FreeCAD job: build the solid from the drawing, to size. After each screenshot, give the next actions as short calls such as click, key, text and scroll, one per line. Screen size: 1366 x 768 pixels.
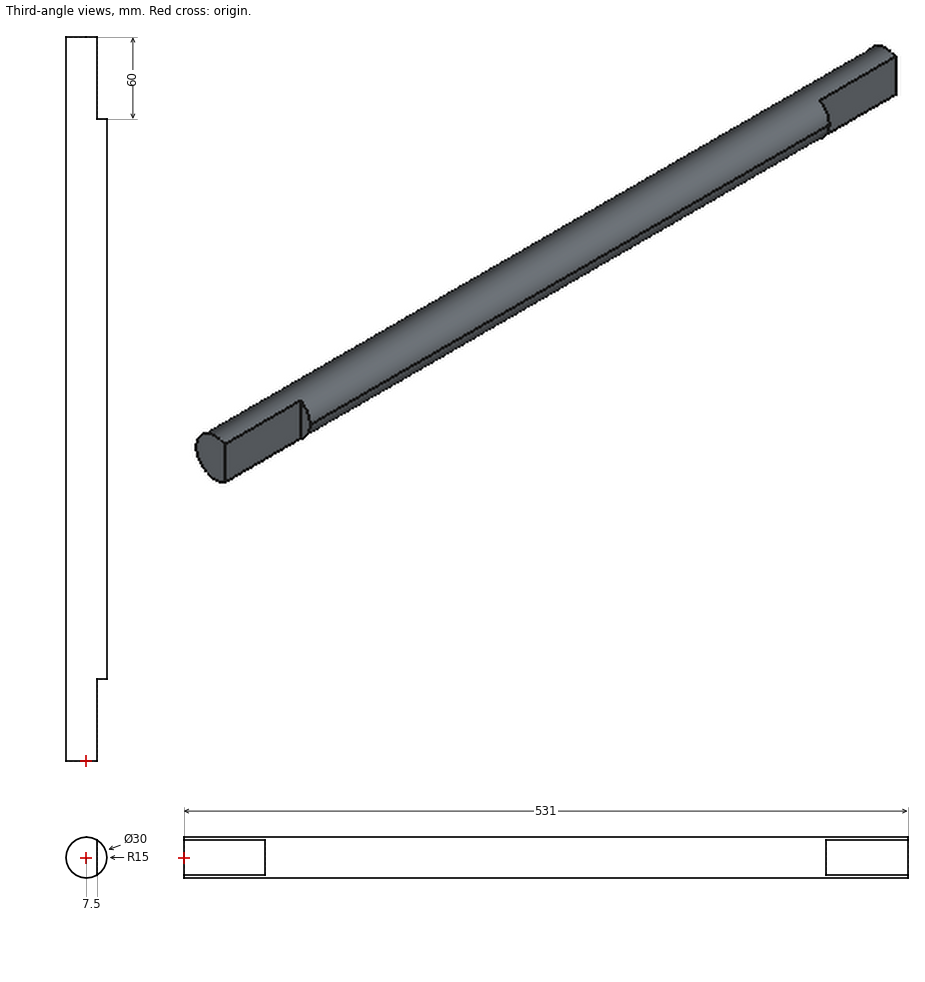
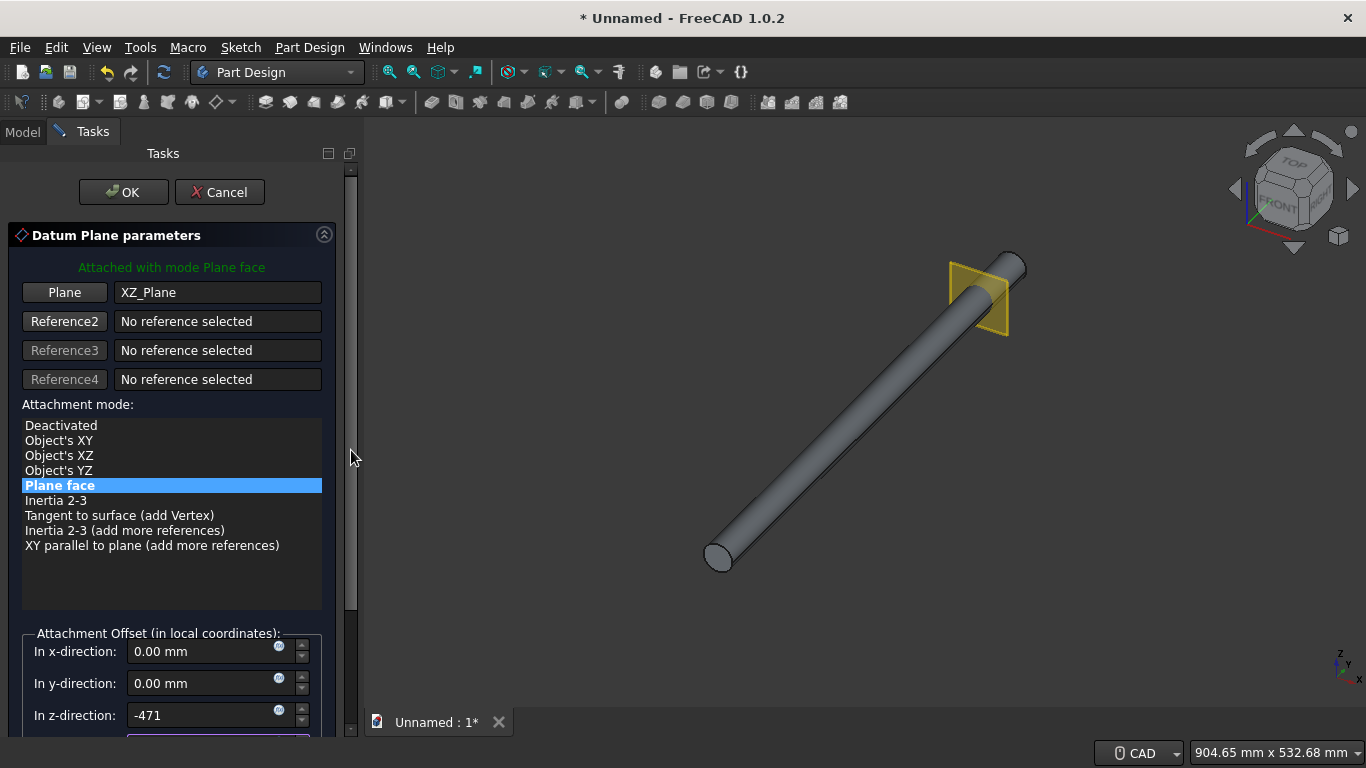
click(124, 192)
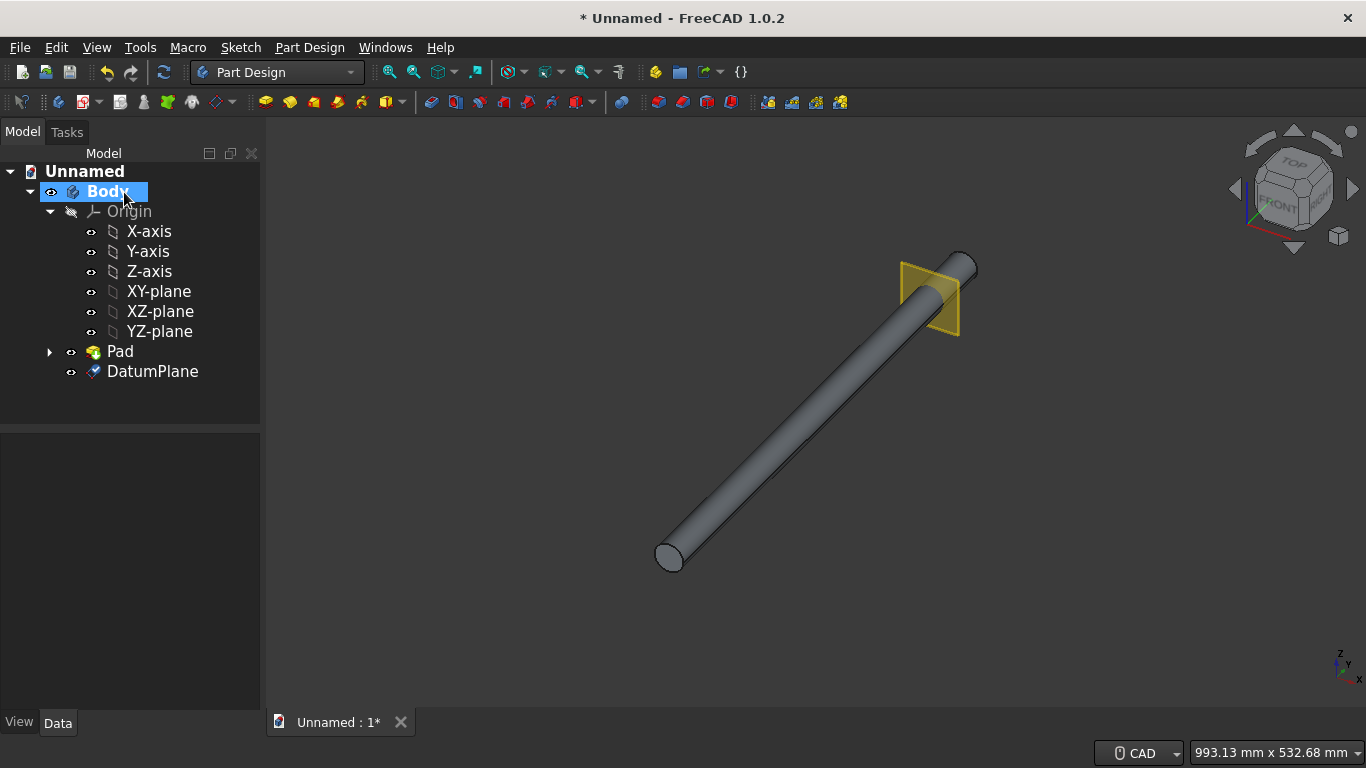
click(116, 372)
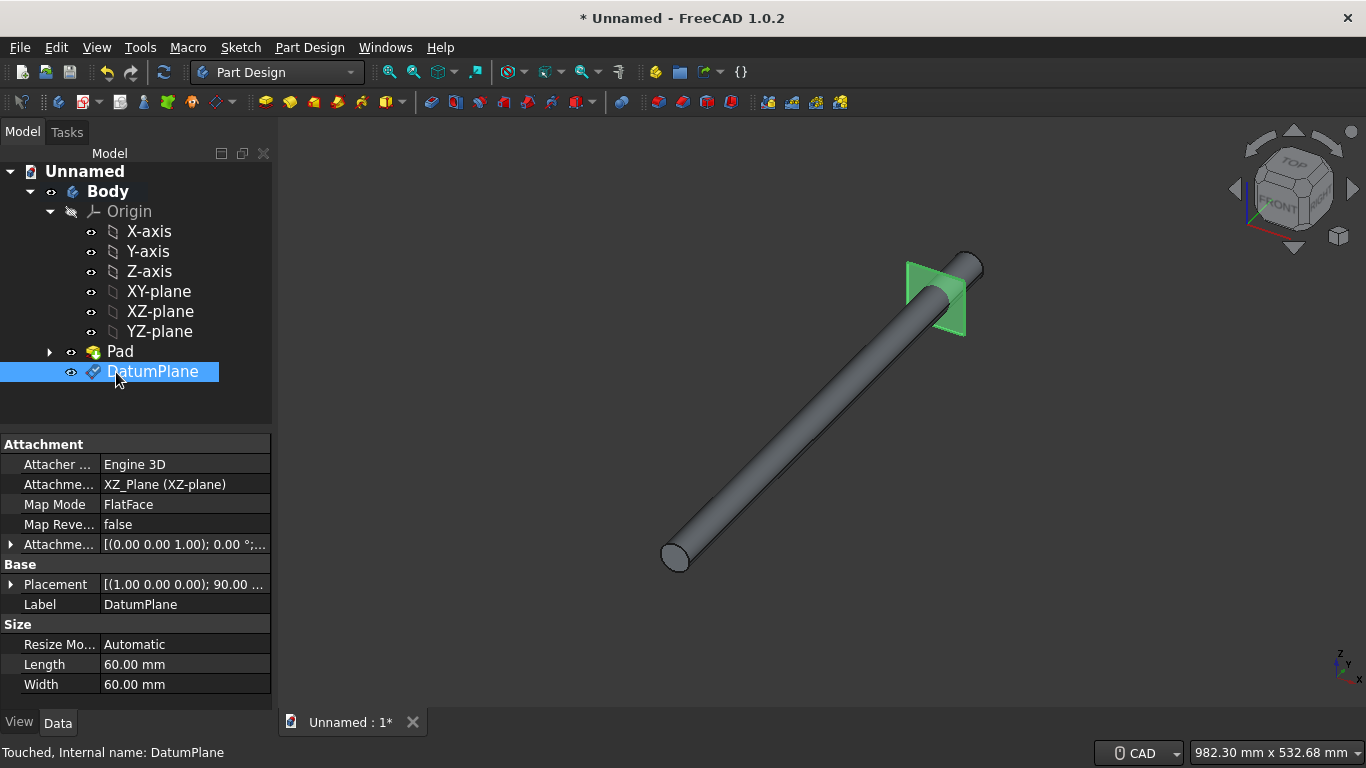
click(84, 102)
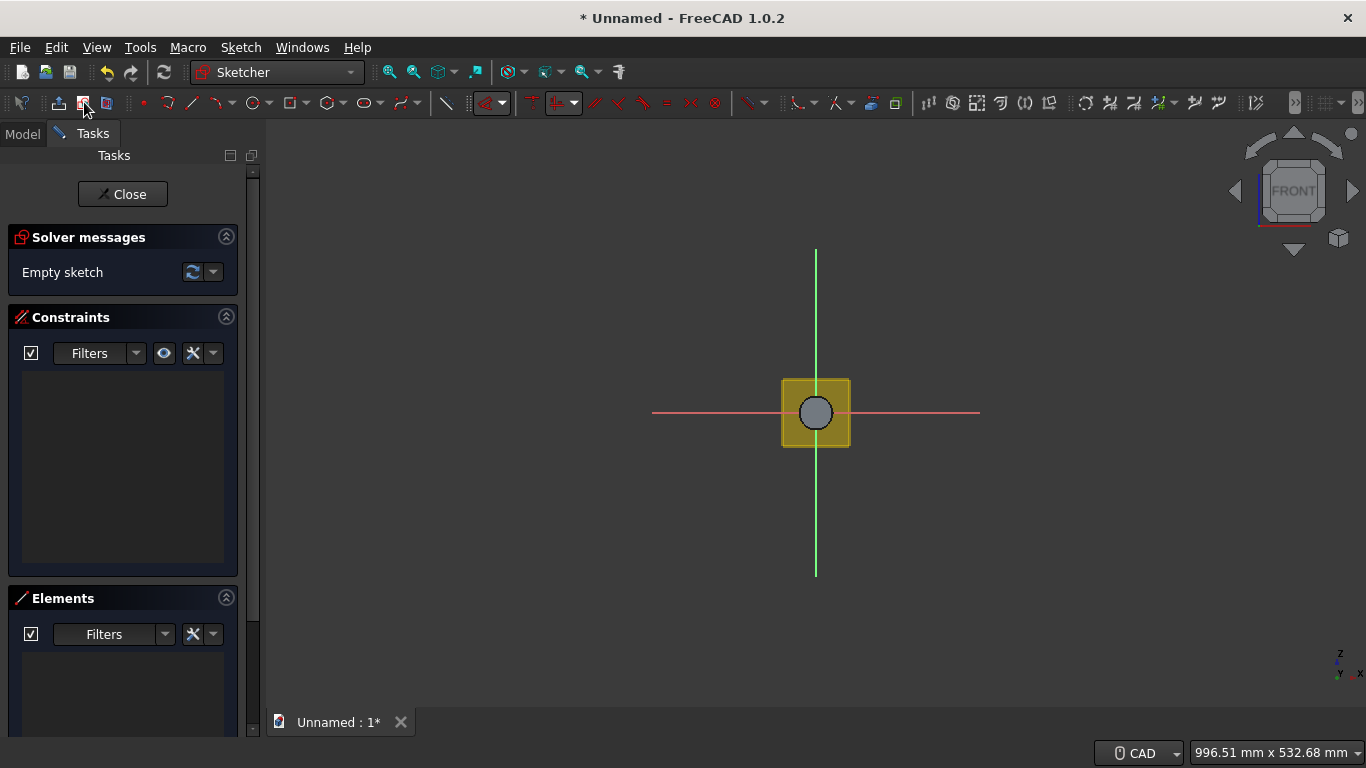
click(108, 104)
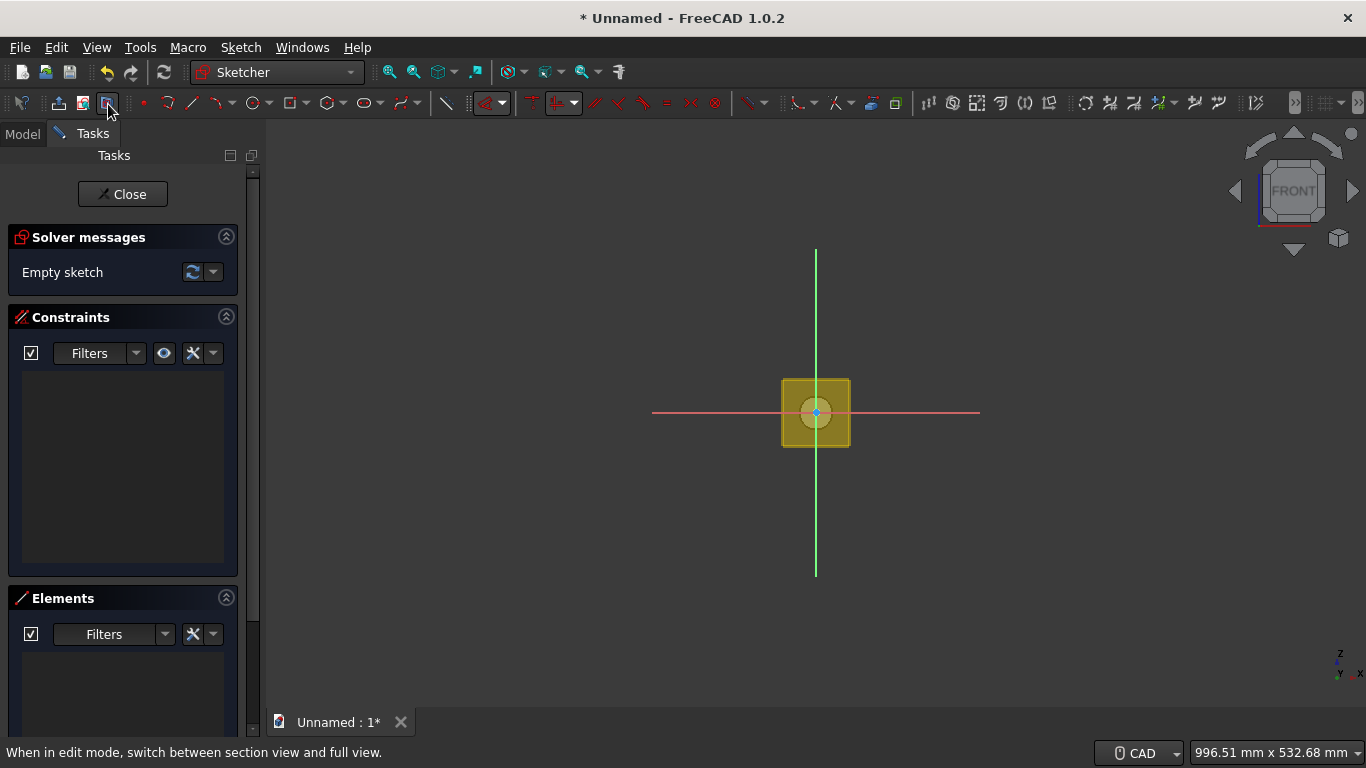
scroll(830, 413, up, 13)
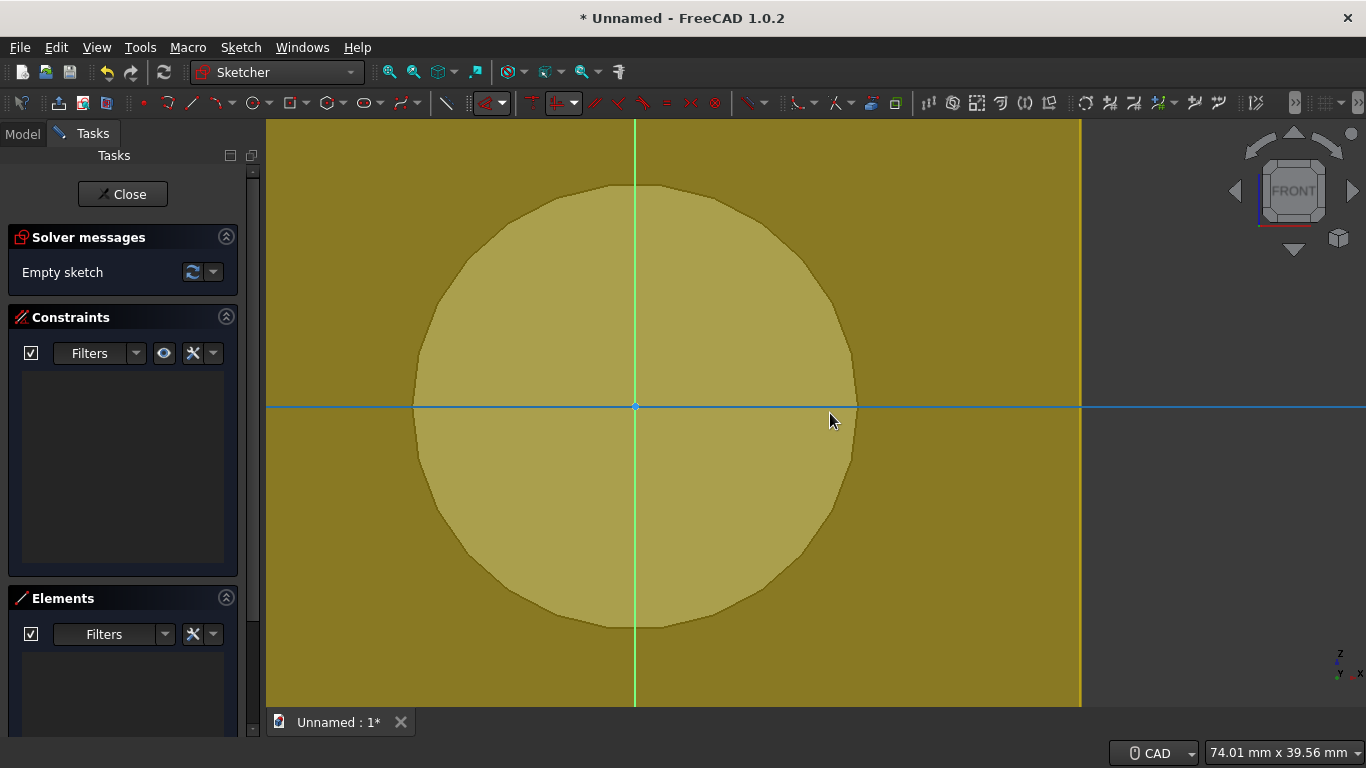
click(192, 104)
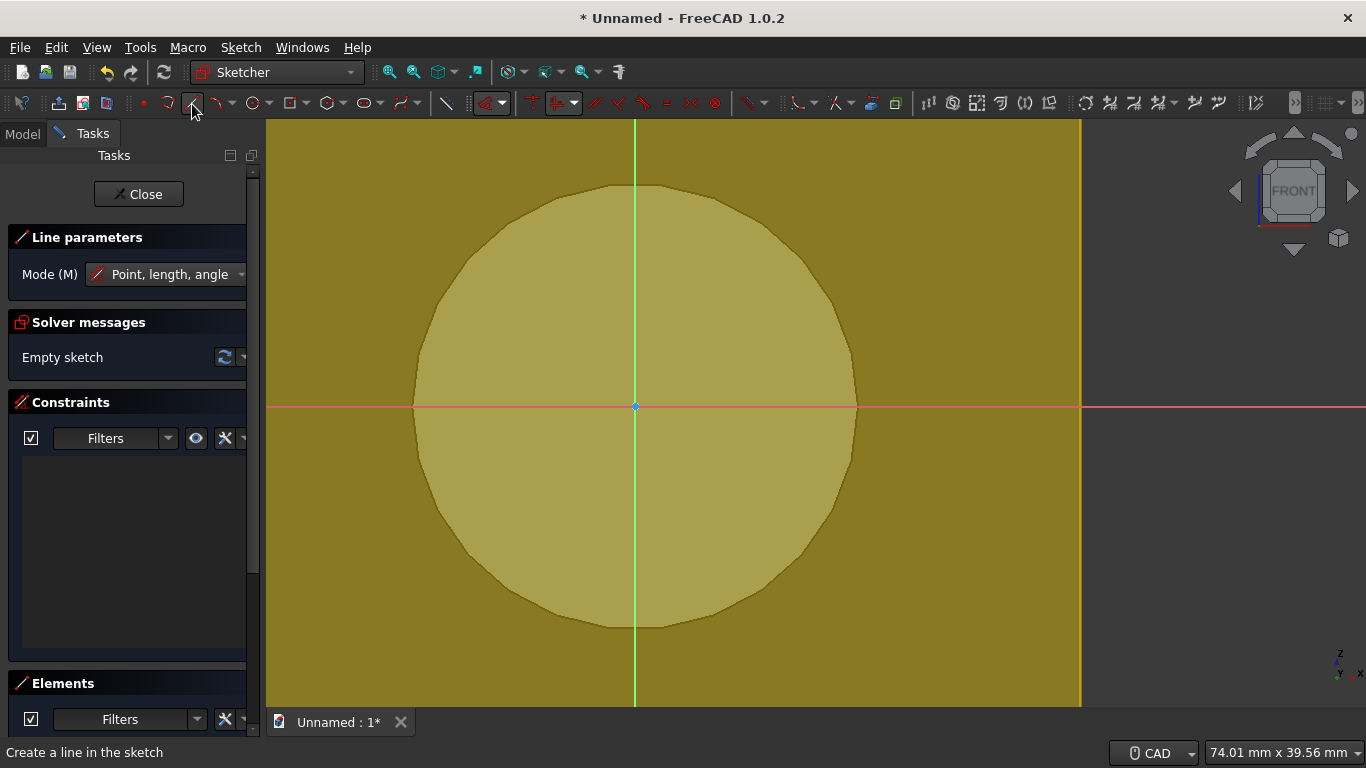
click(747, 600)
click(747, 214)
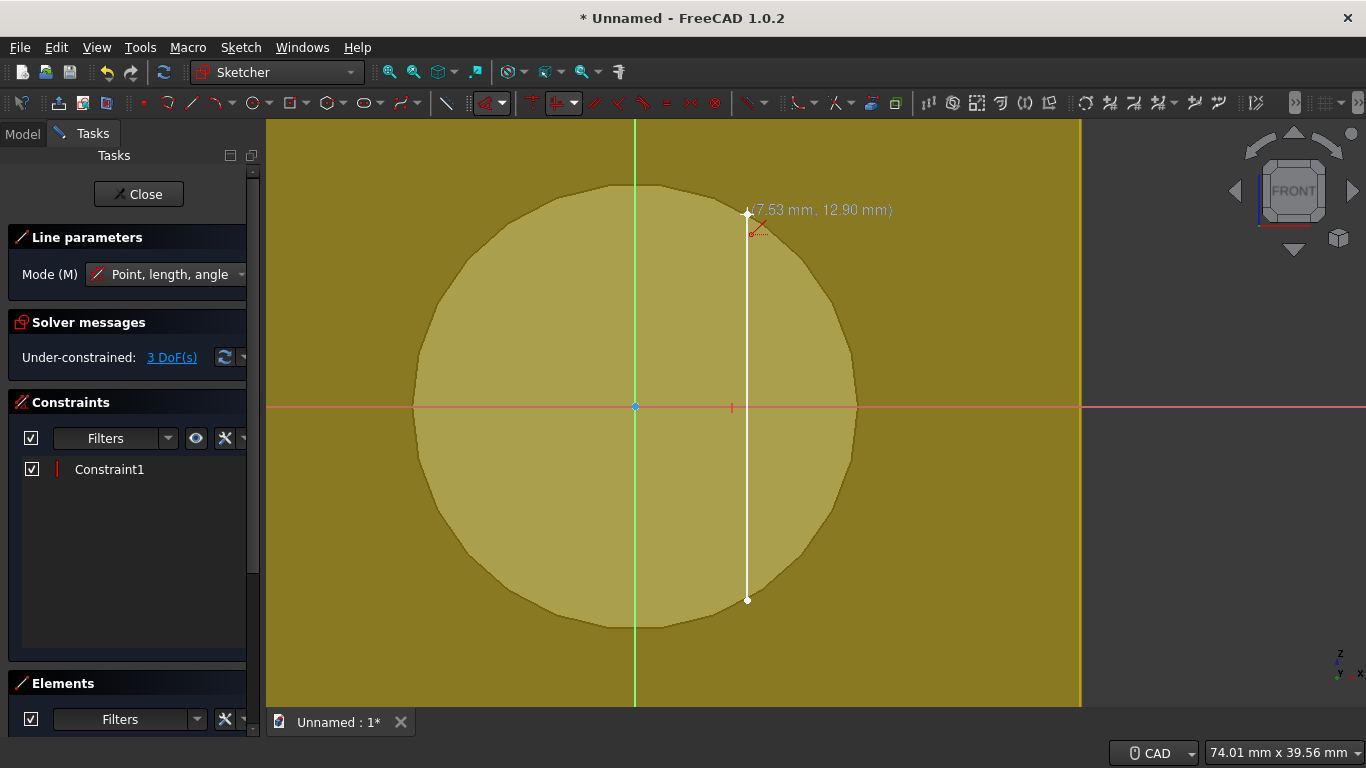
key(g)
key(3)
key(a)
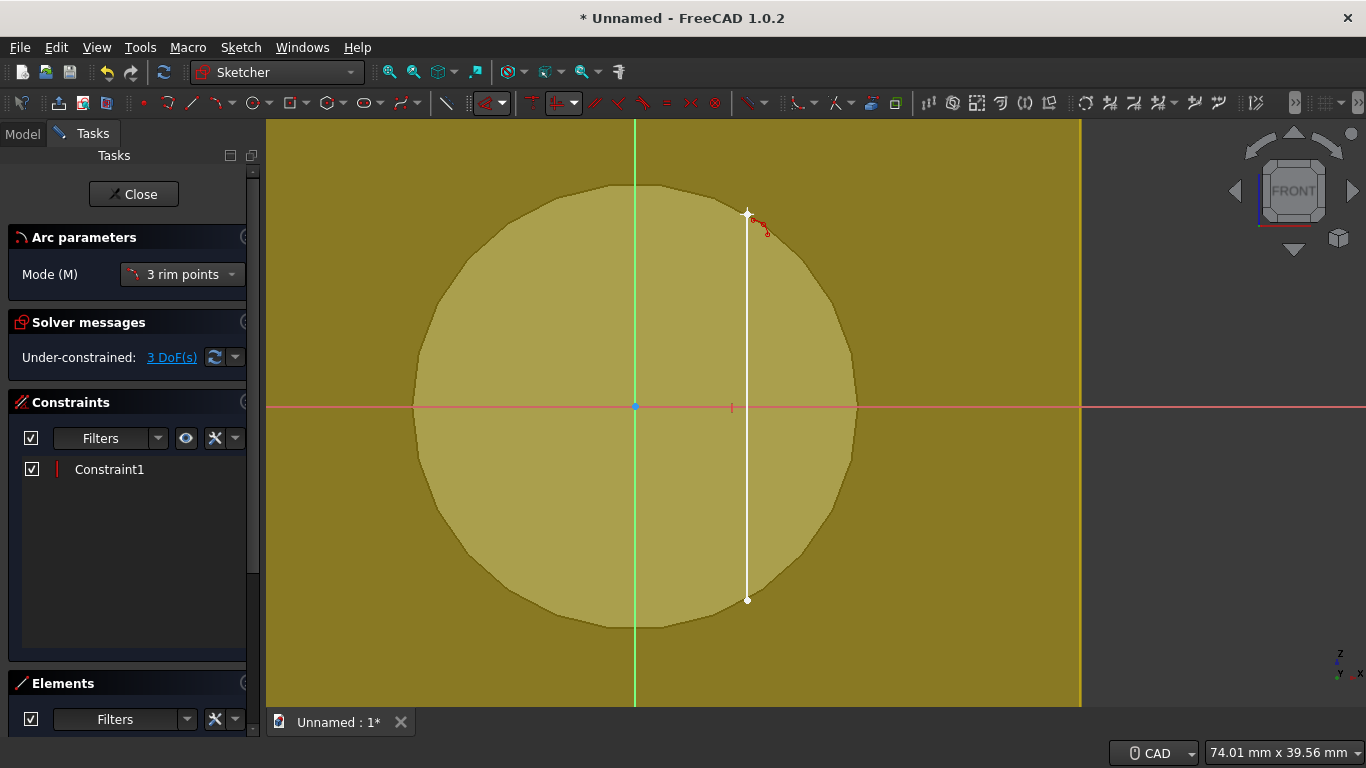
click(747, 215)
click(747, 601)
click(853, 453)
key(Escape)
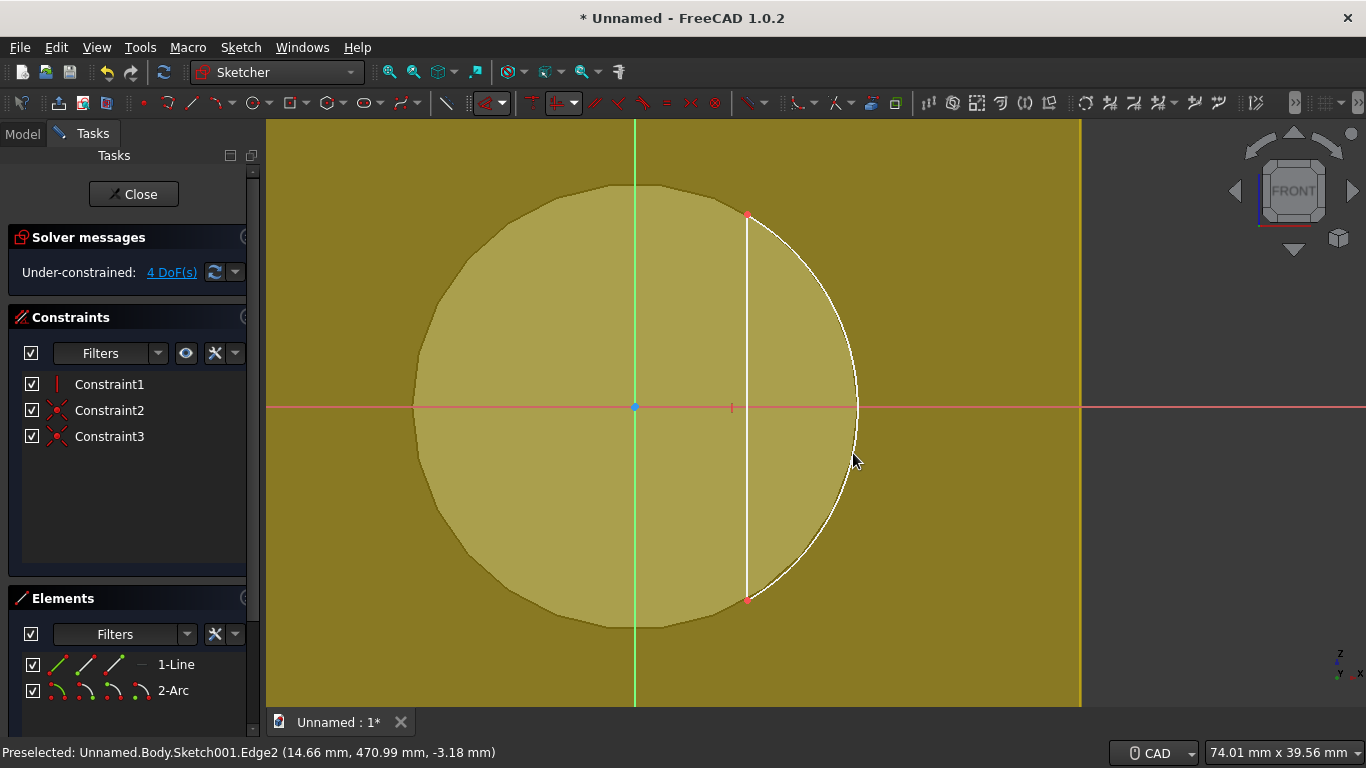
drag(624, 397, 645, 418)